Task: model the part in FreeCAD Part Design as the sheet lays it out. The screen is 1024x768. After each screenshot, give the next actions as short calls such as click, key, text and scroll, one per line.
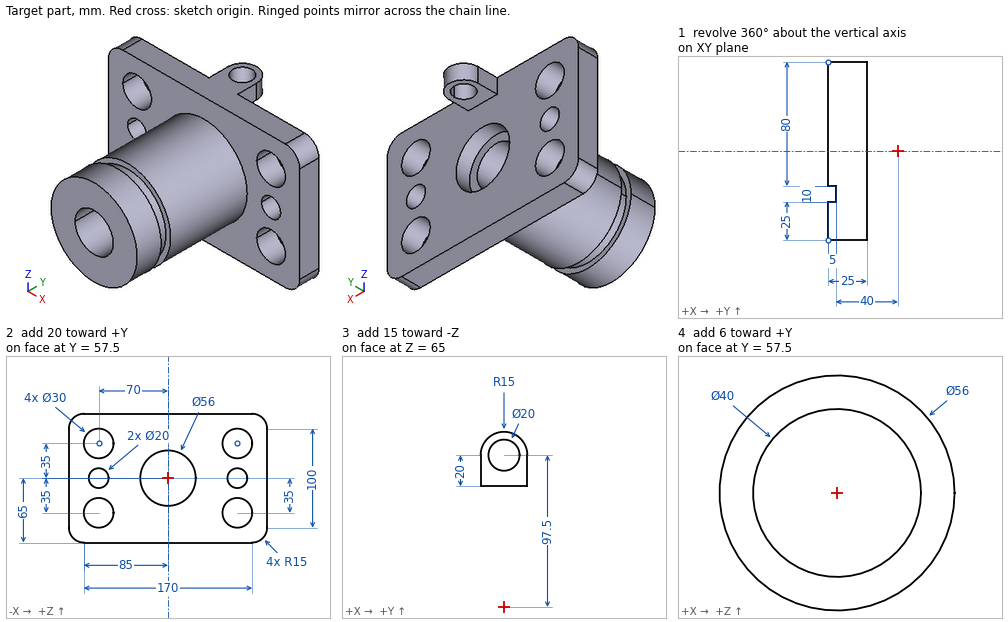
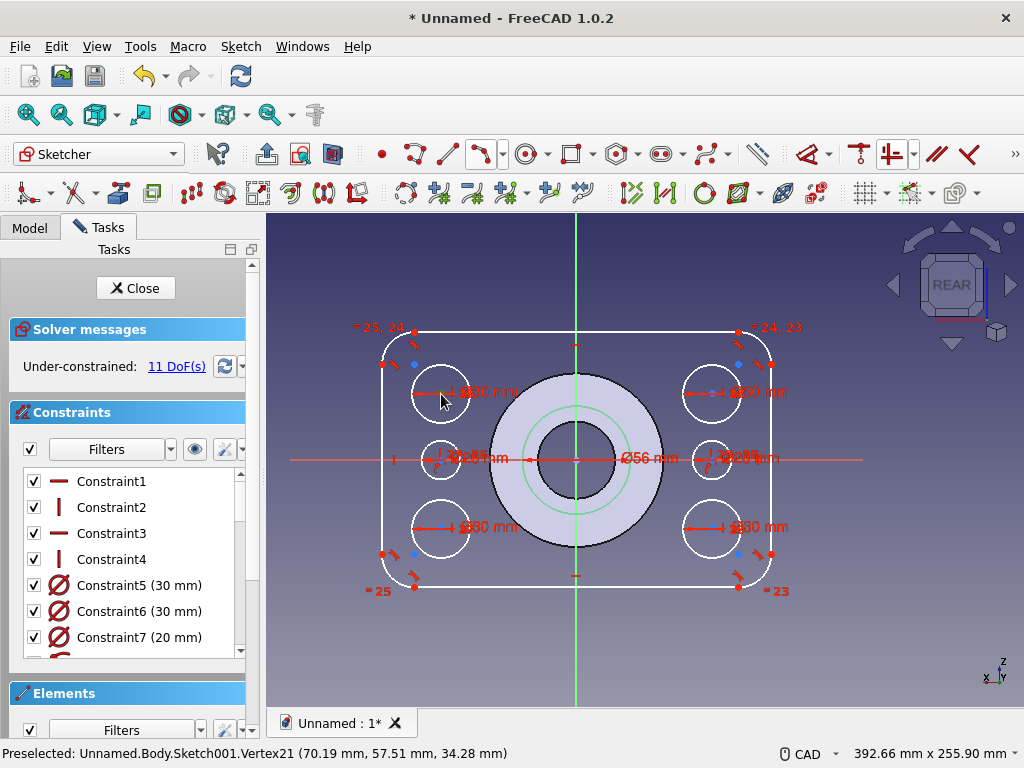
click(712, 394)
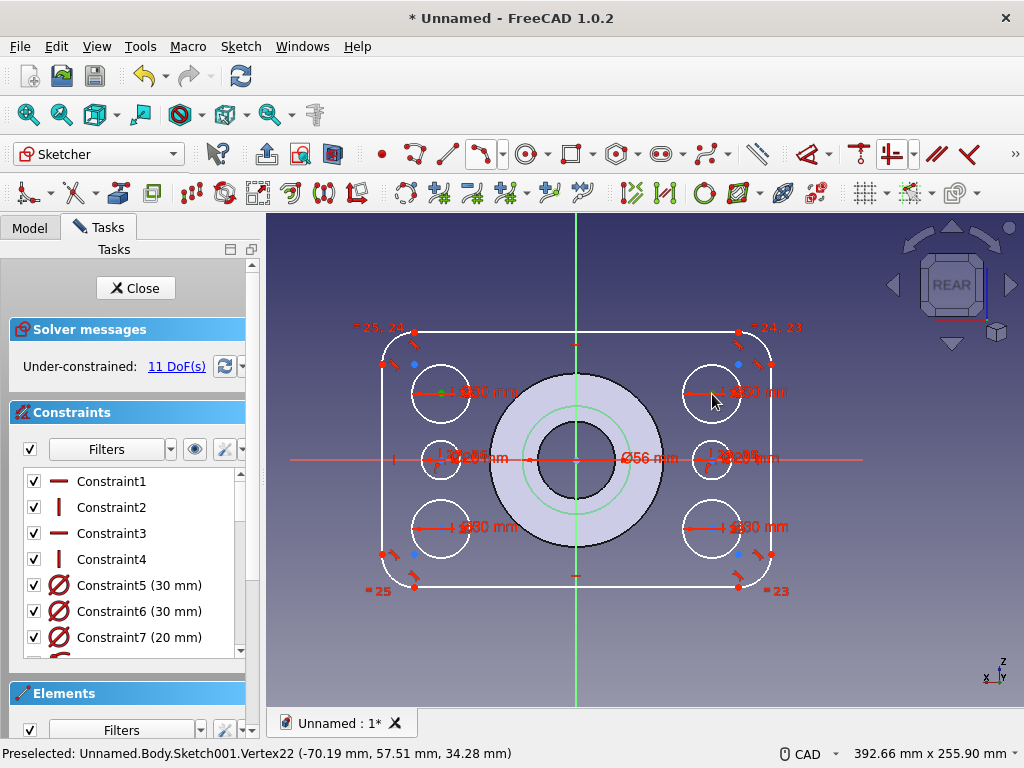
click(577, 648)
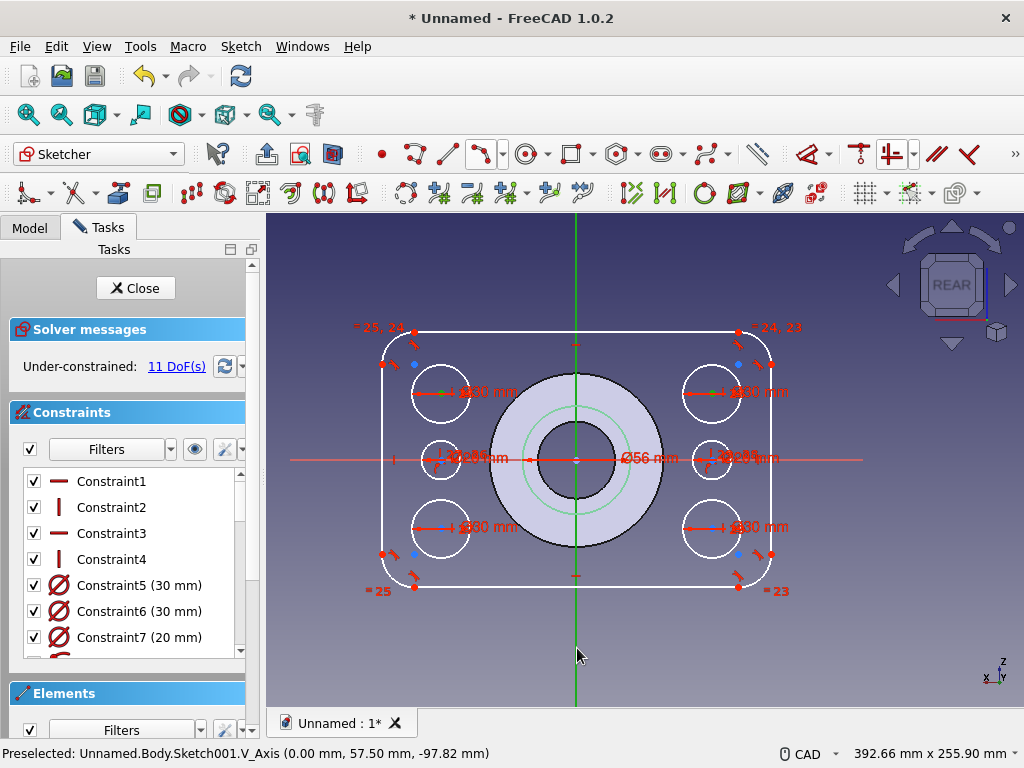
key(s)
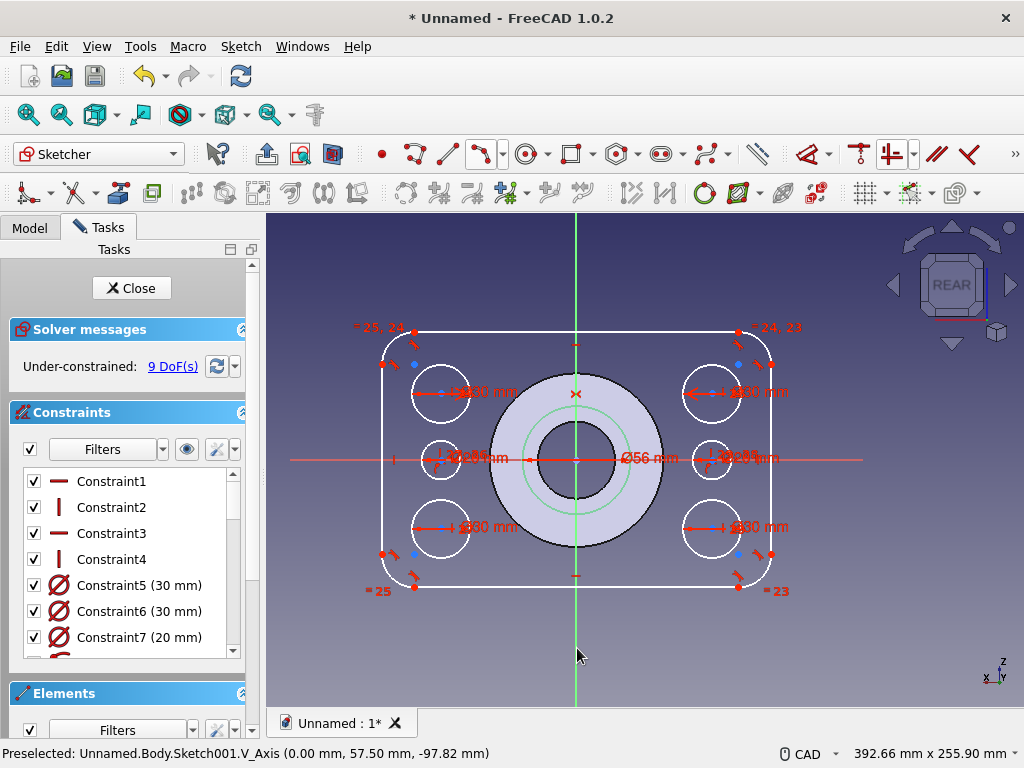
click(806, 154)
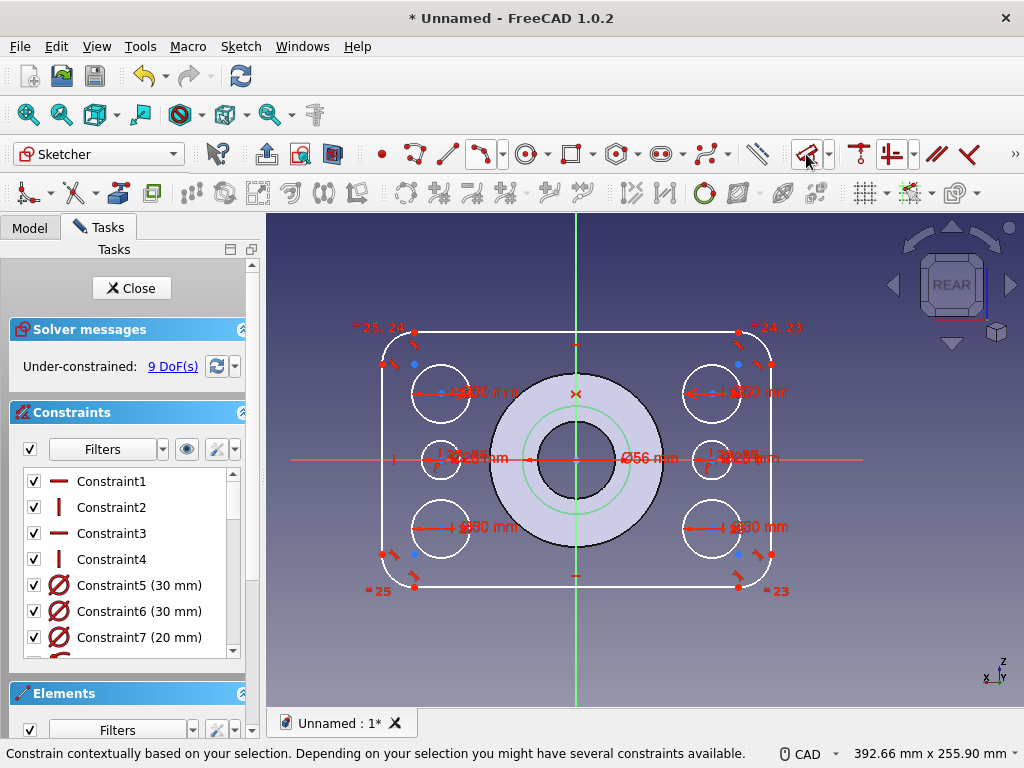
scroll(753, 584, up, 2)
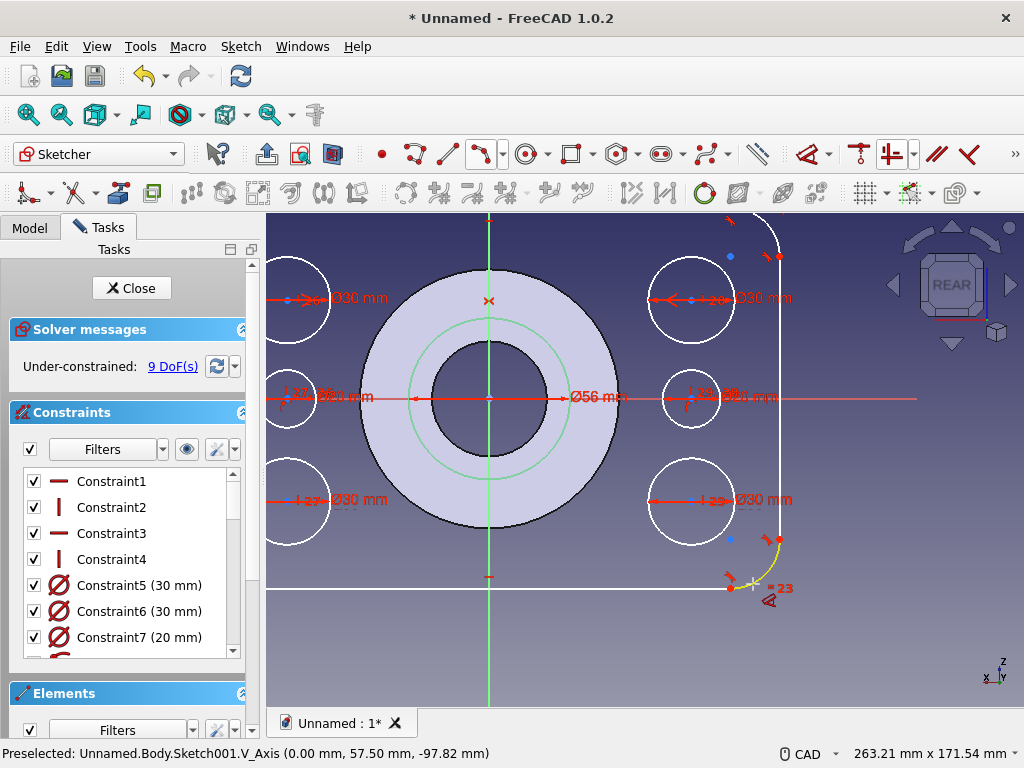
click(753, 583)
click(768, 611)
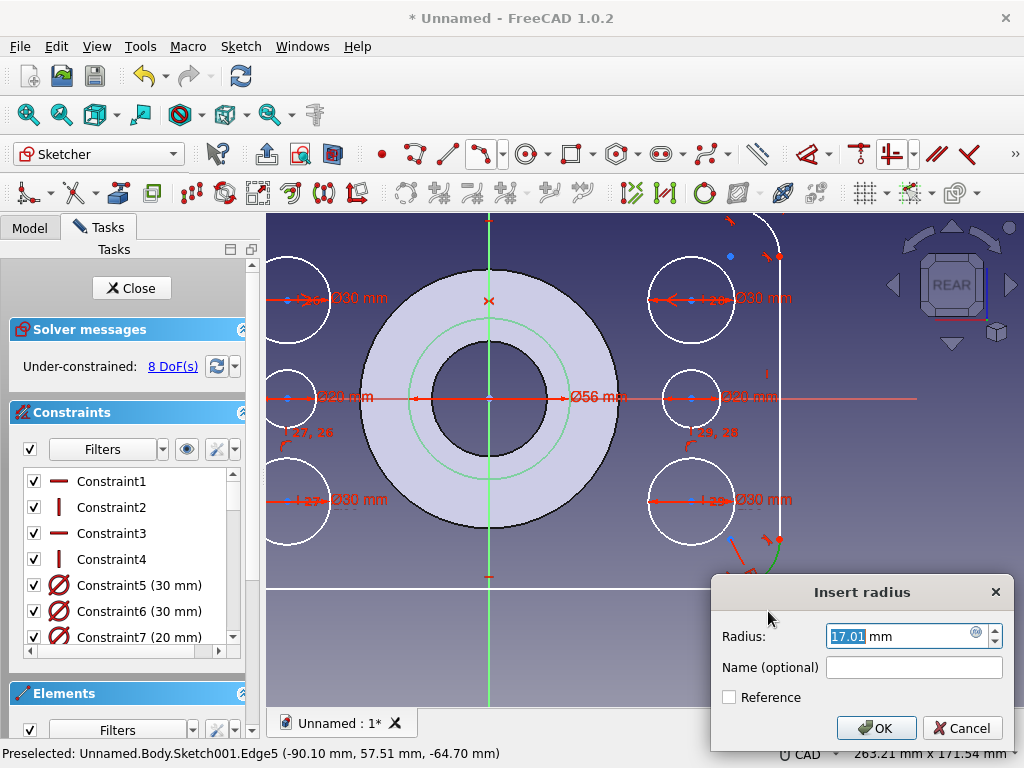
text(15)
key(Return)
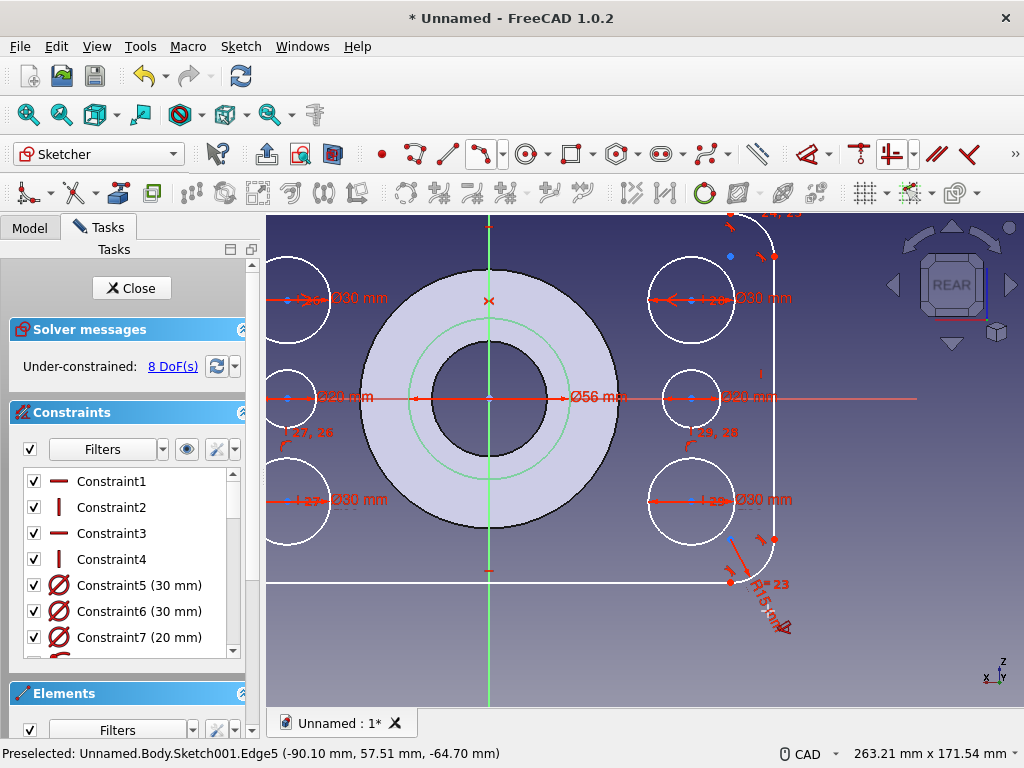
scroll(754, 584, down, 2)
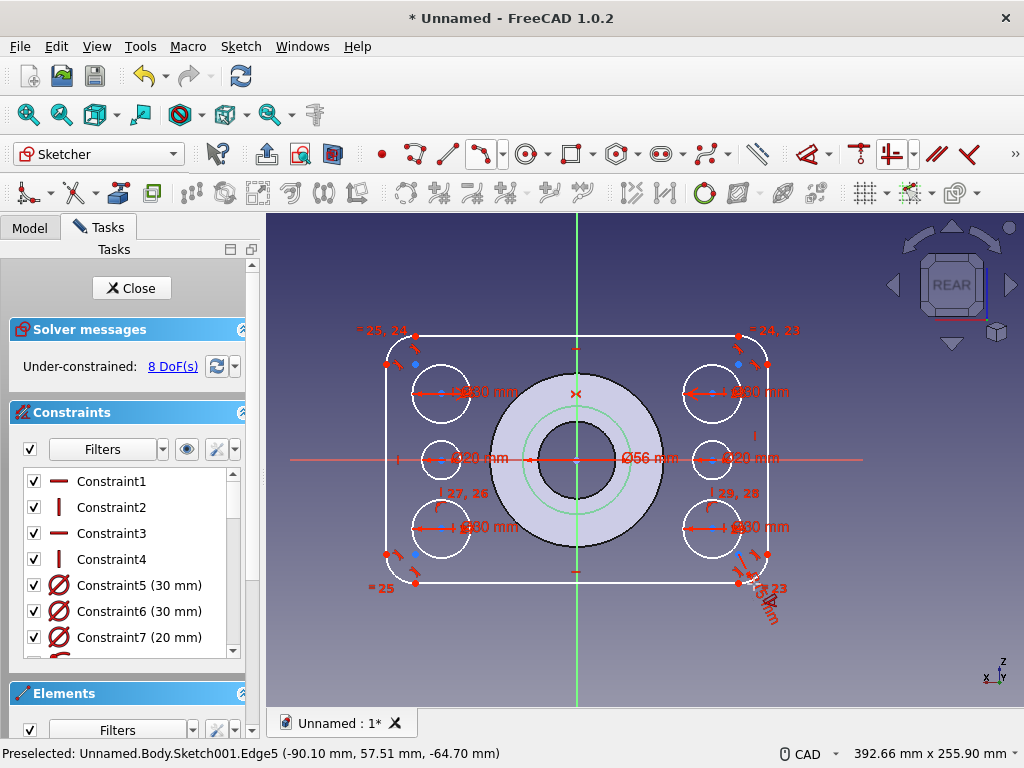
click(441, 394)
click(509, 360)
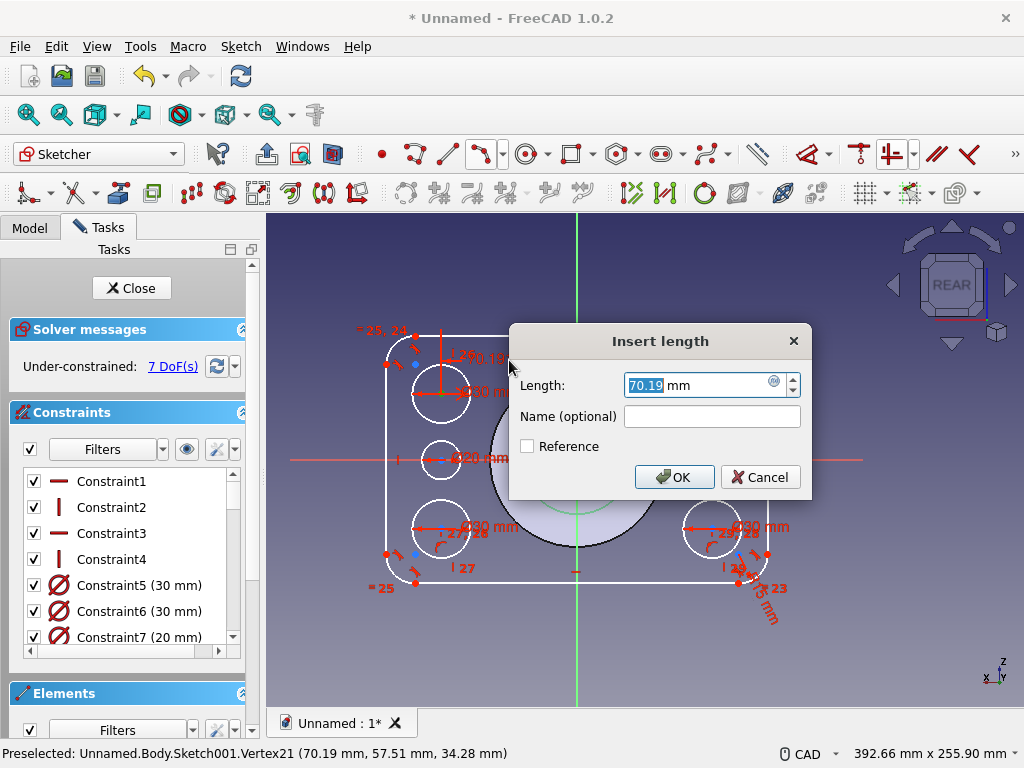
text(70)
key(Return)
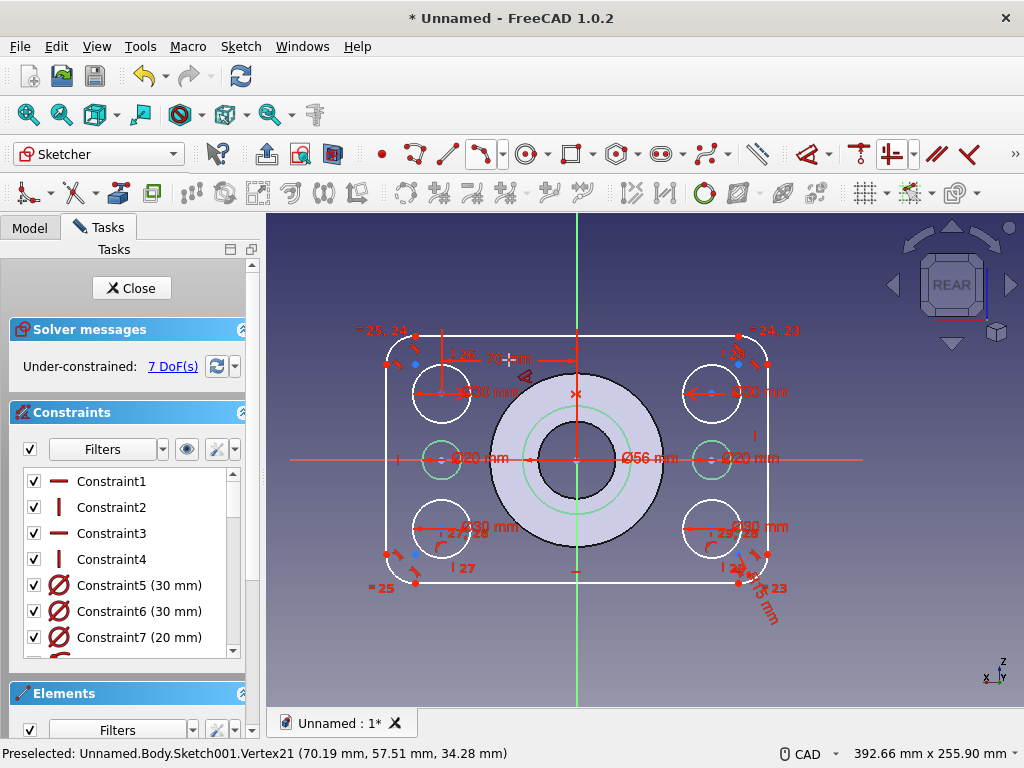
click(442, 394)
click(408, 427)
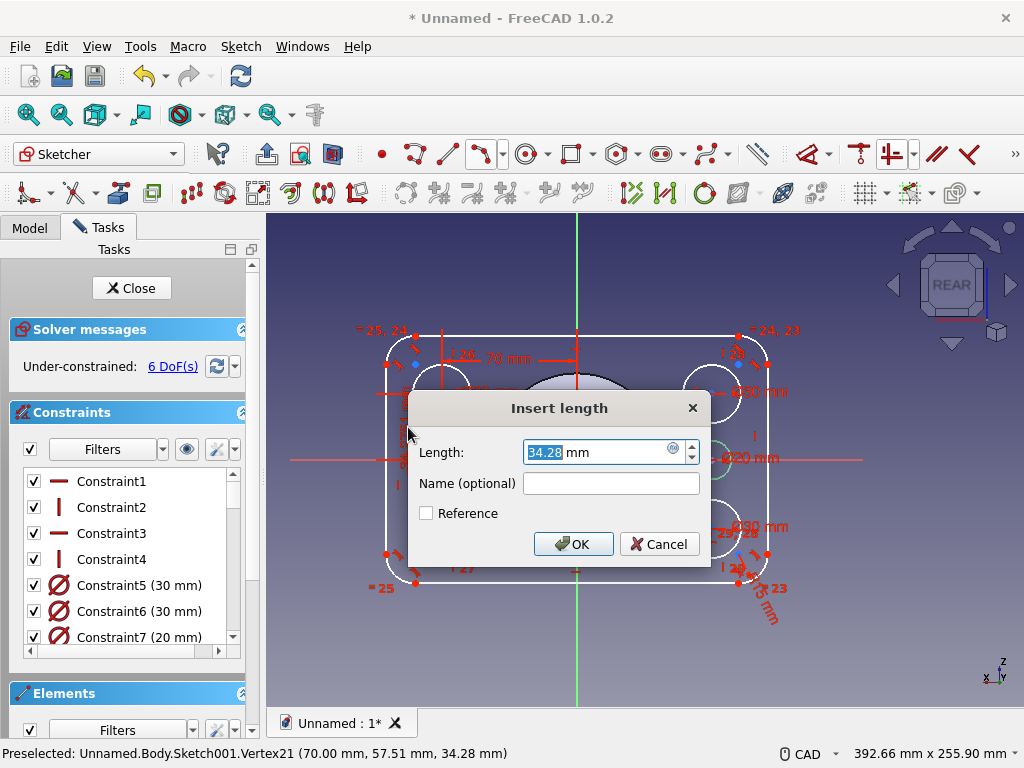
text(35)
key(Return)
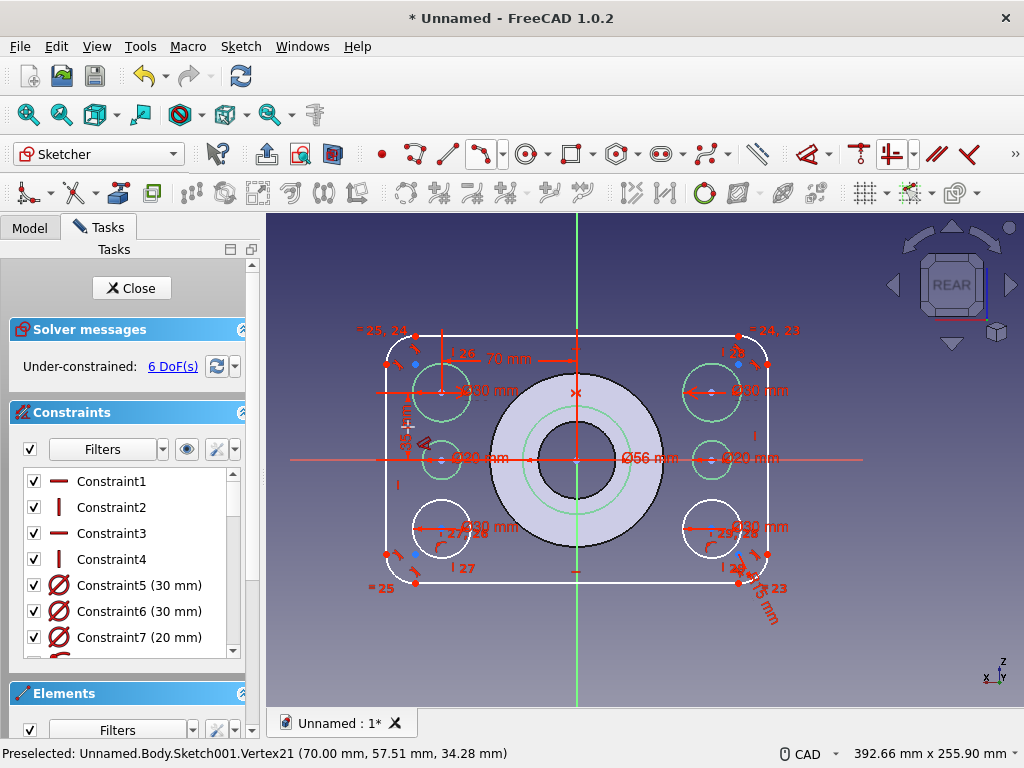
click(442, 529)
click(408, 495)